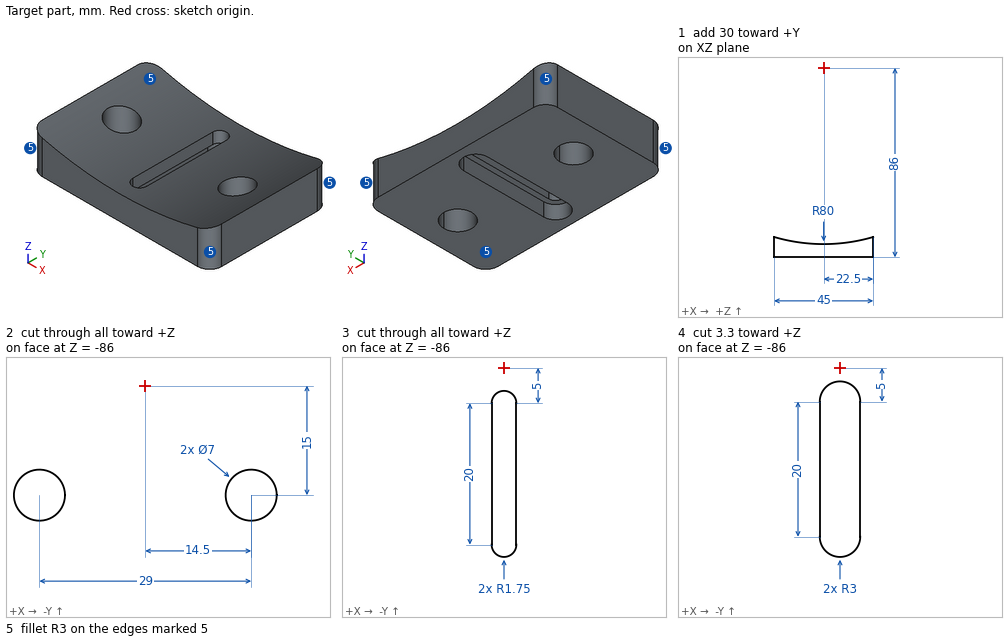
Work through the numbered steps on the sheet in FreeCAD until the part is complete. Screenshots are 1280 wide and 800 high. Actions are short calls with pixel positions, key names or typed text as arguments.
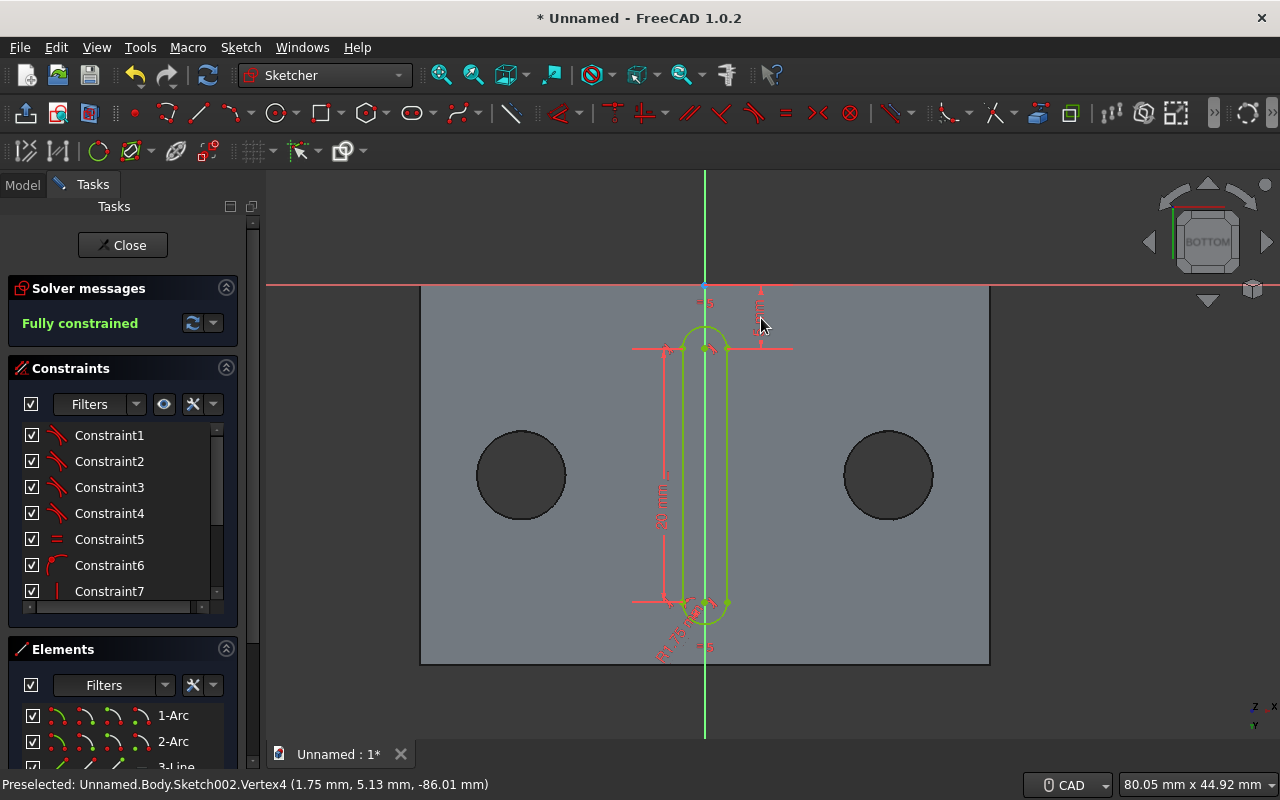
click(123, 245)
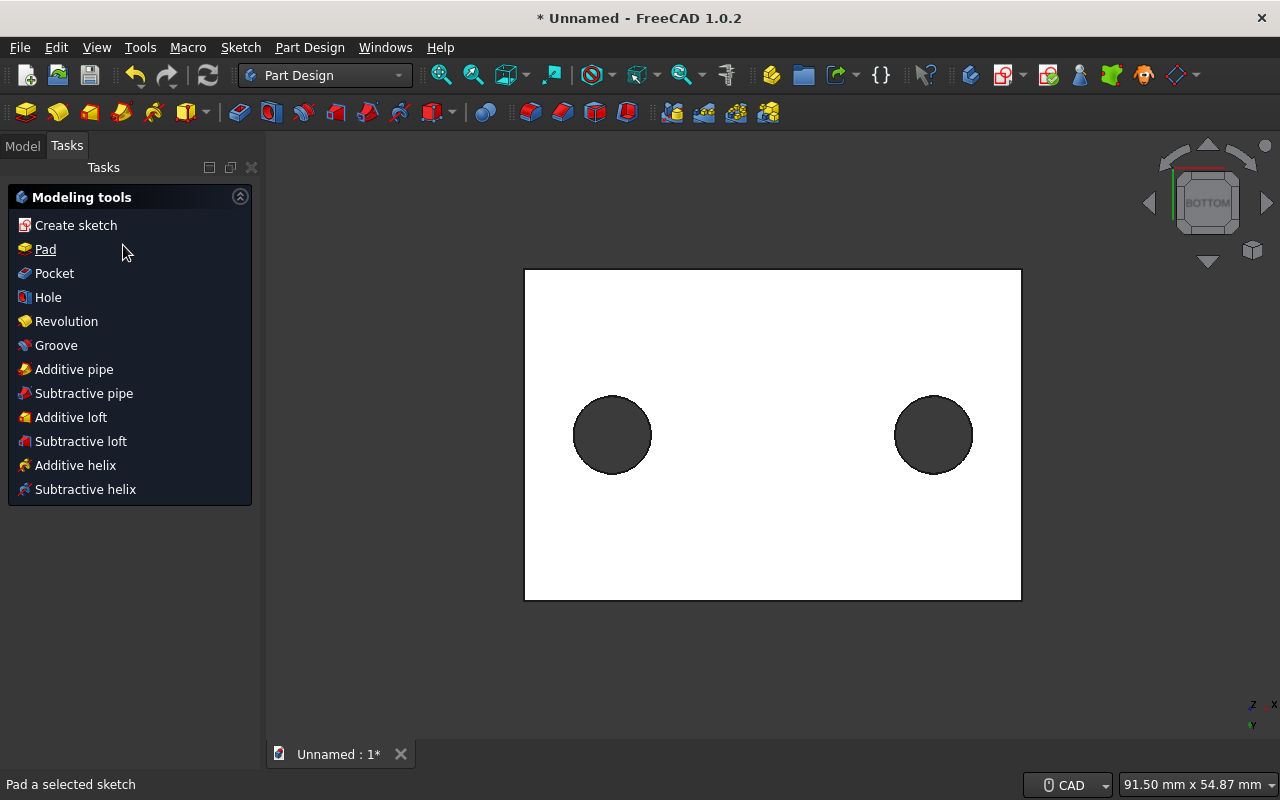
click(240, 112)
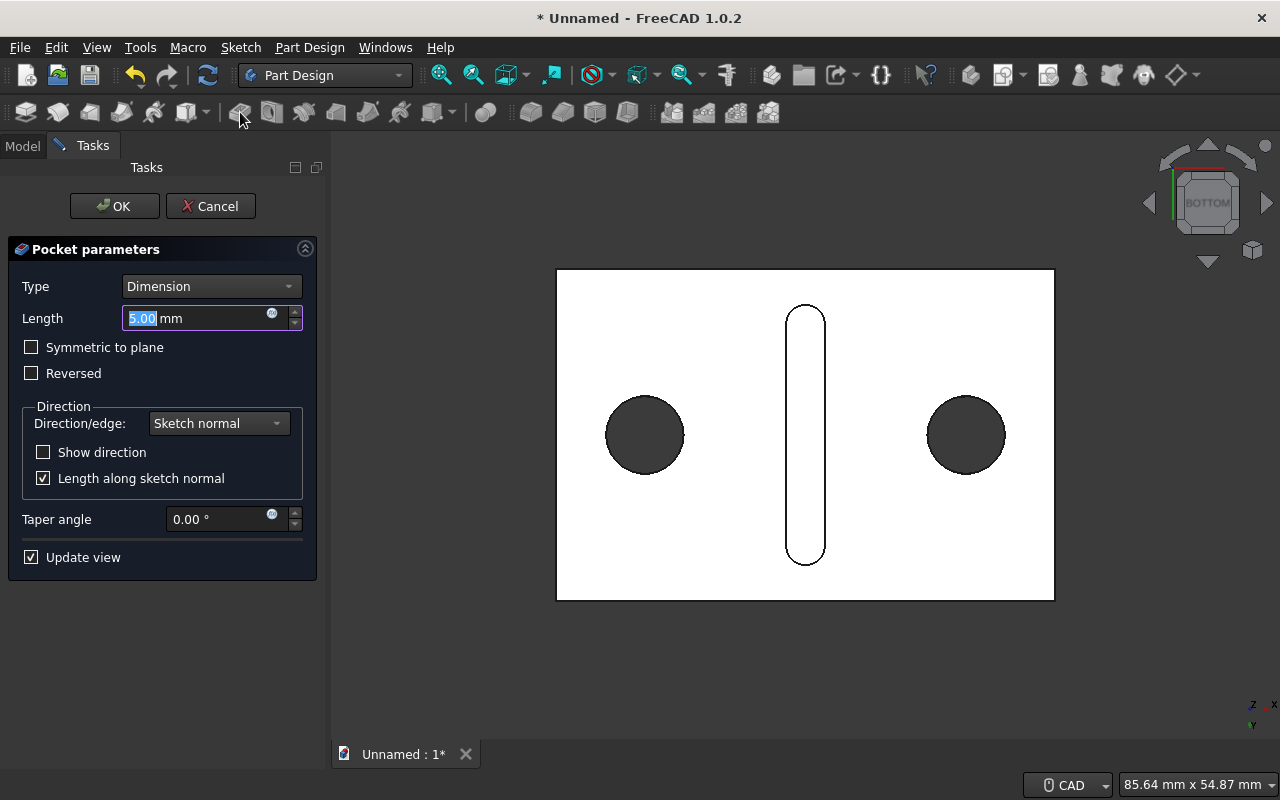
click(212, 286)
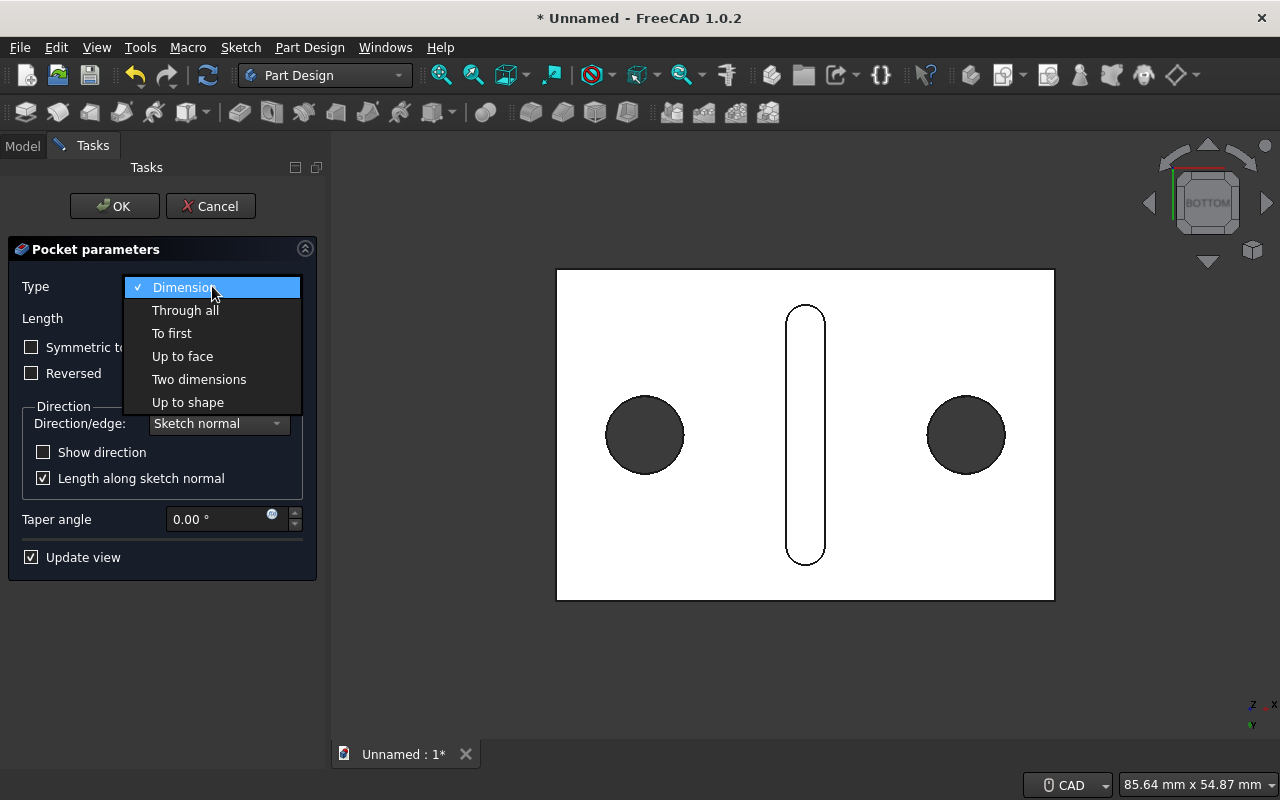
click(212, 310)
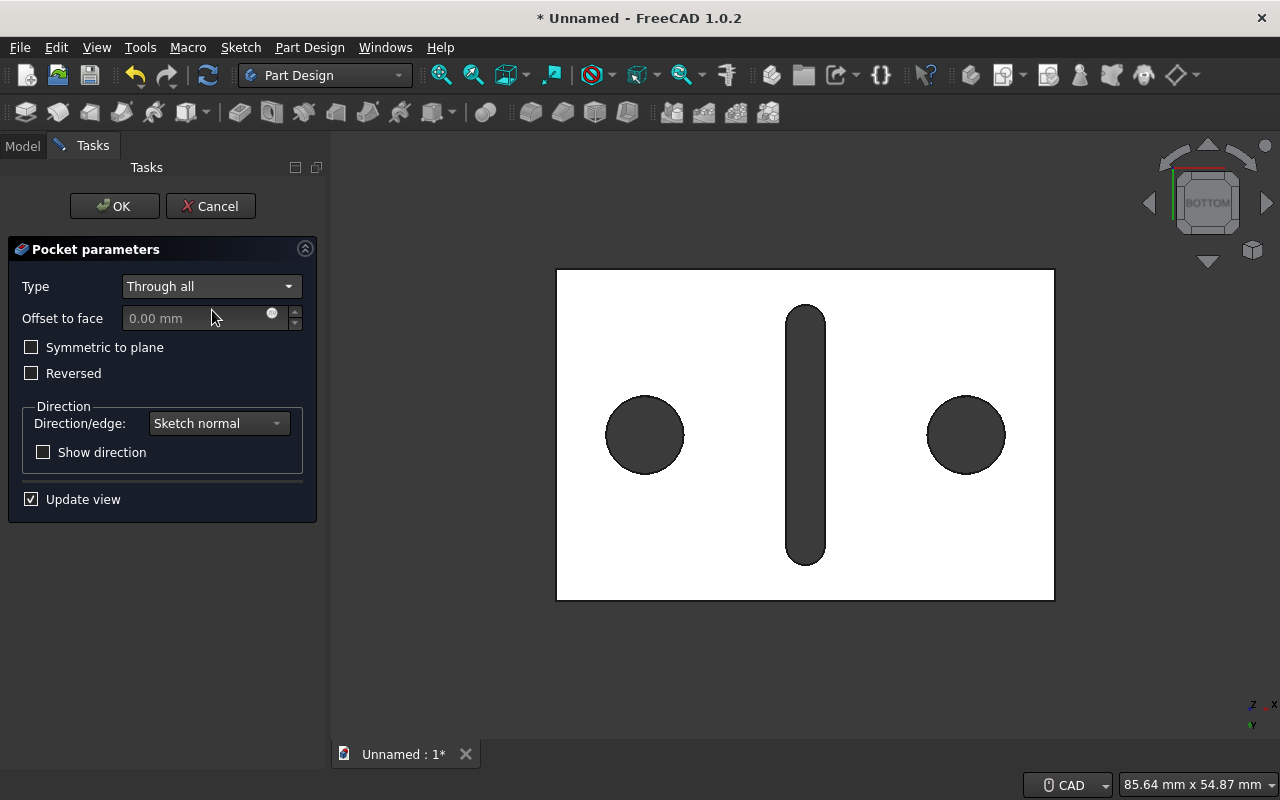
click(115, 206)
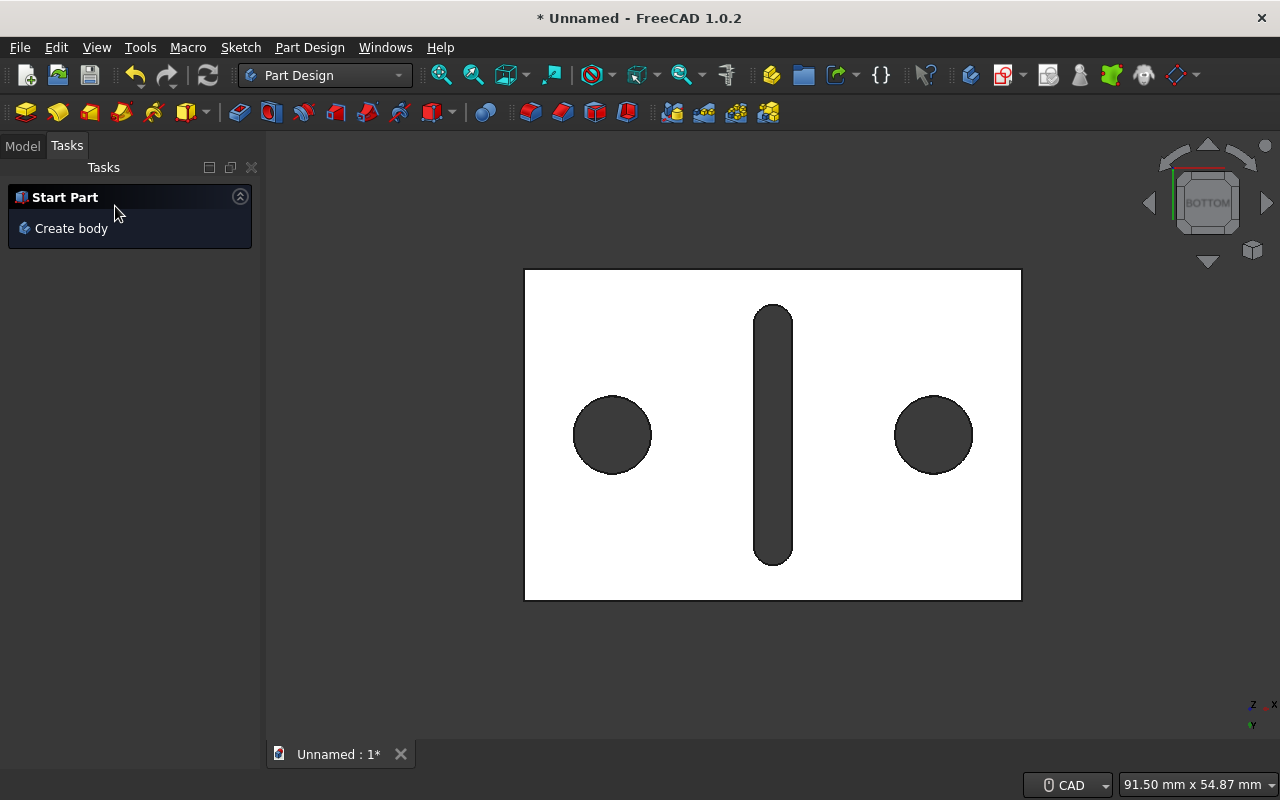
click(631, 339)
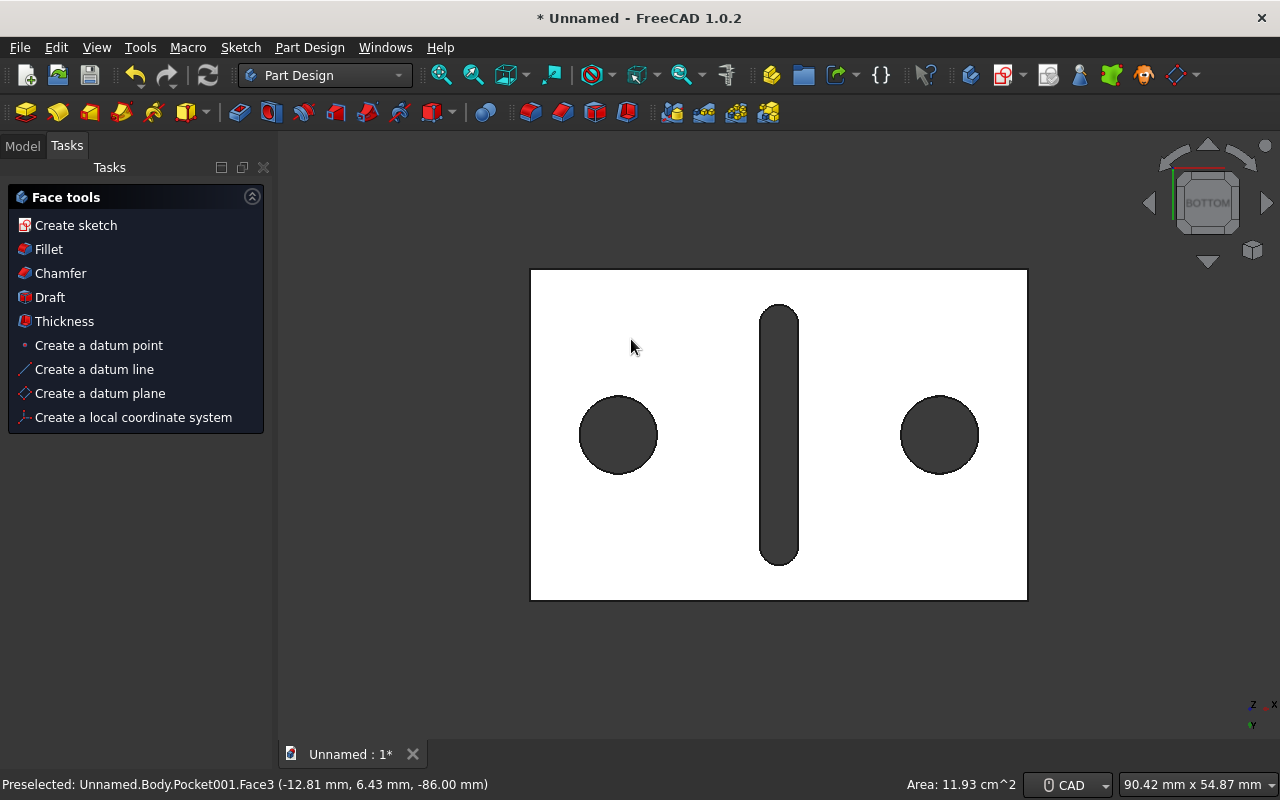
click(1004, 76)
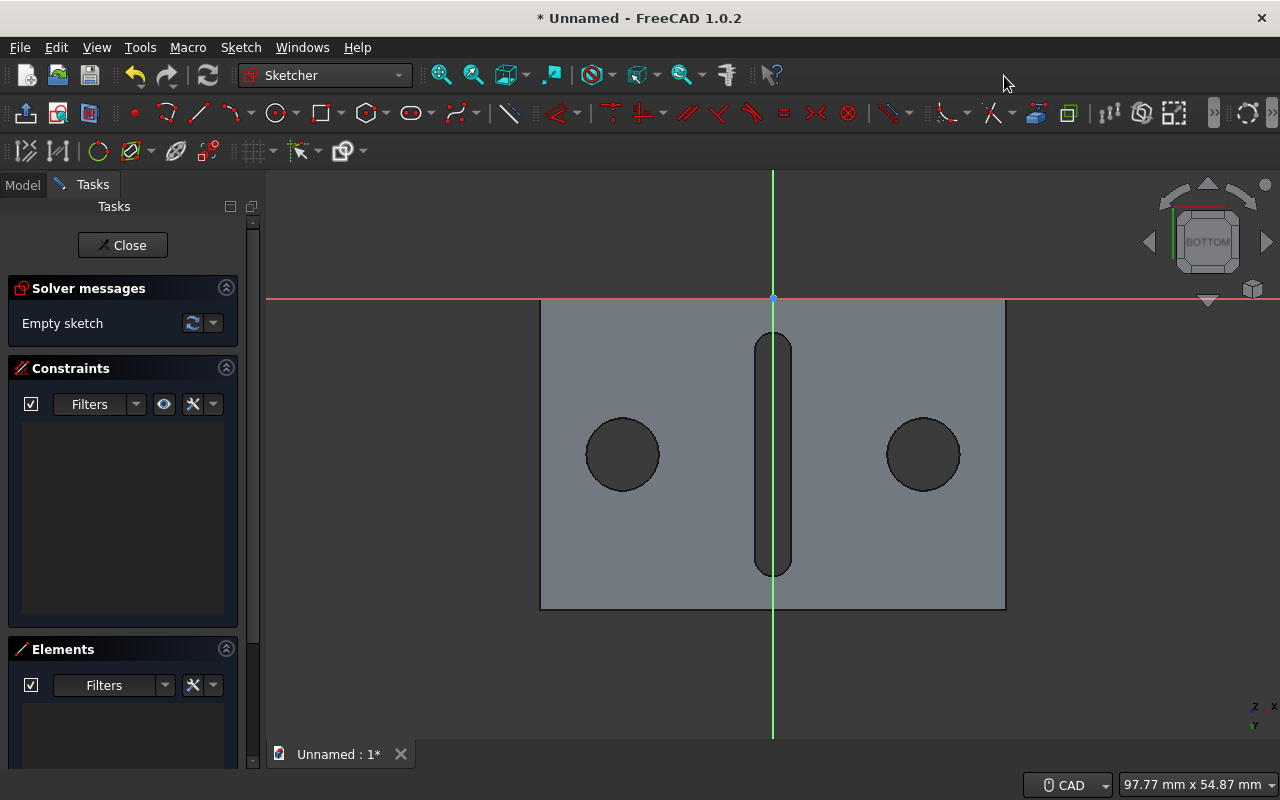
click(412, 114)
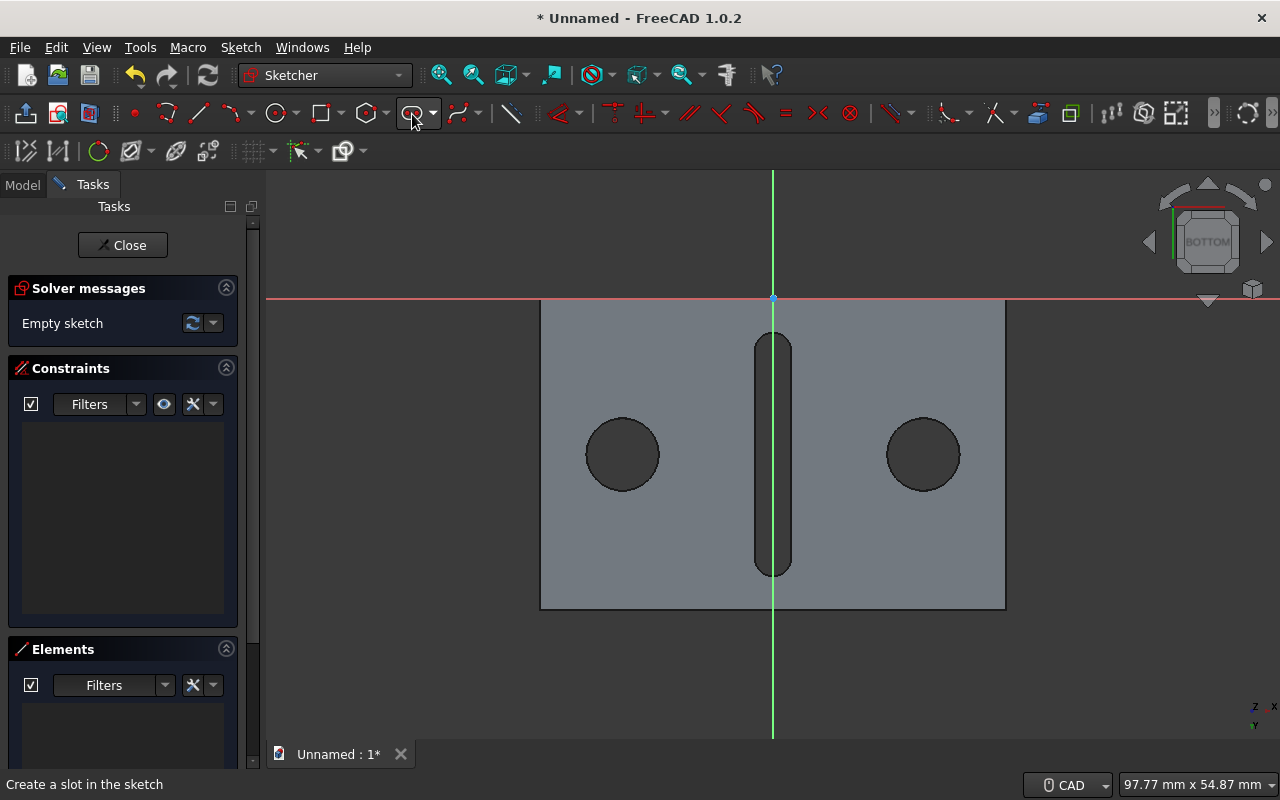
click(773, 558)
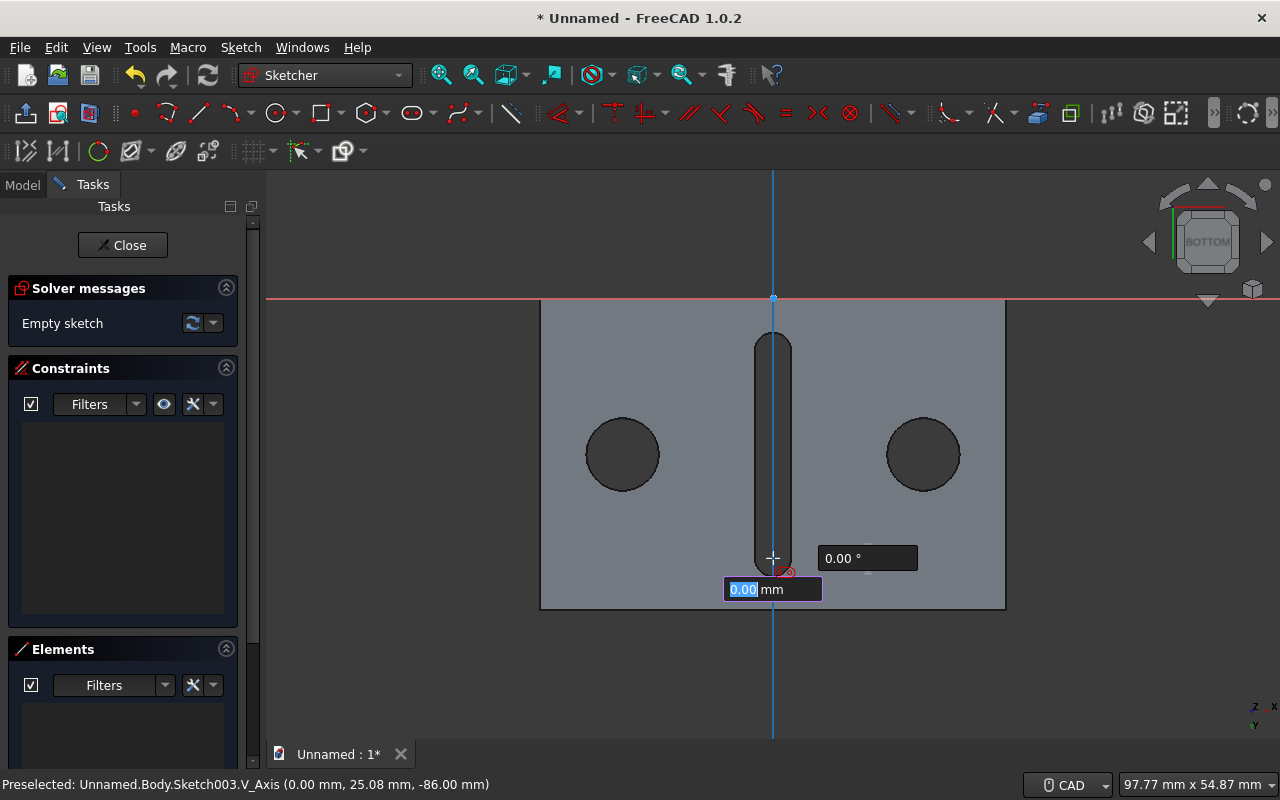
click(782, 351)